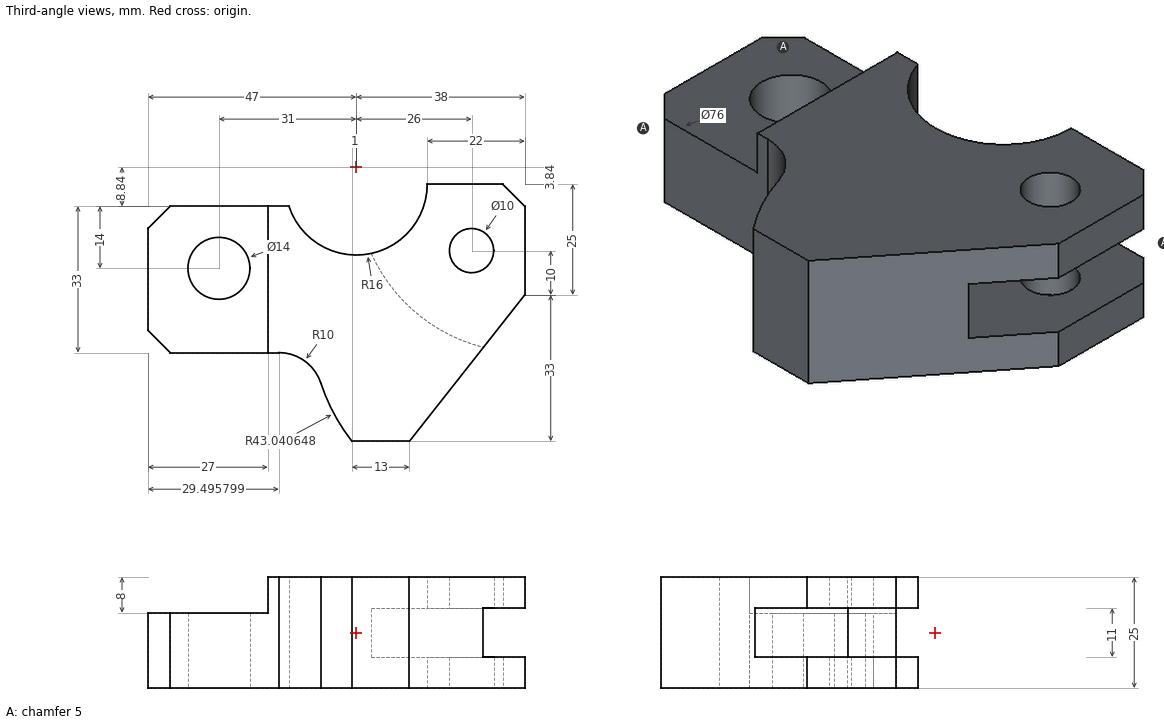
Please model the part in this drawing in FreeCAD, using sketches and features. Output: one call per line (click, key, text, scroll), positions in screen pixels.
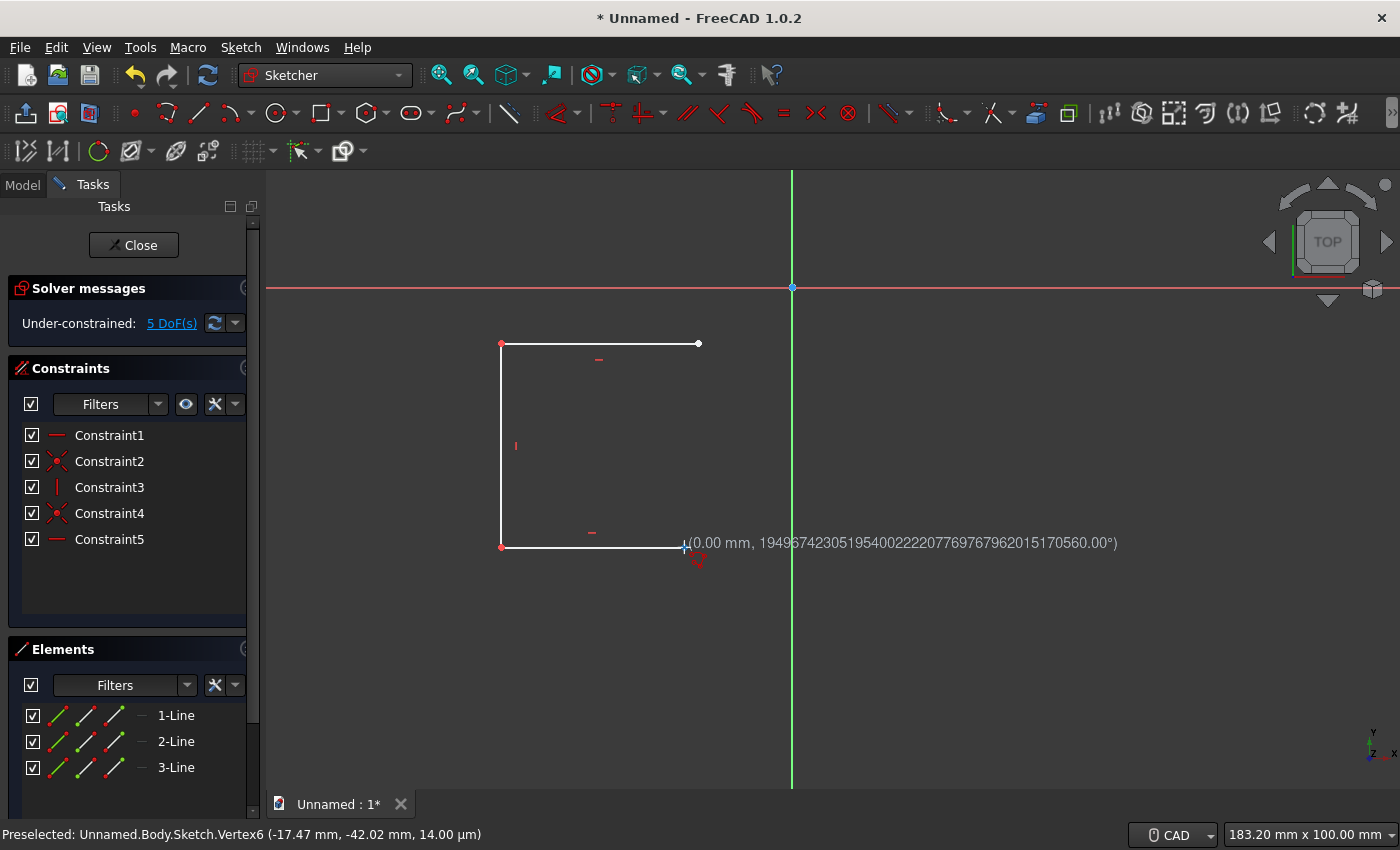
scroll(786, 671, up, 5)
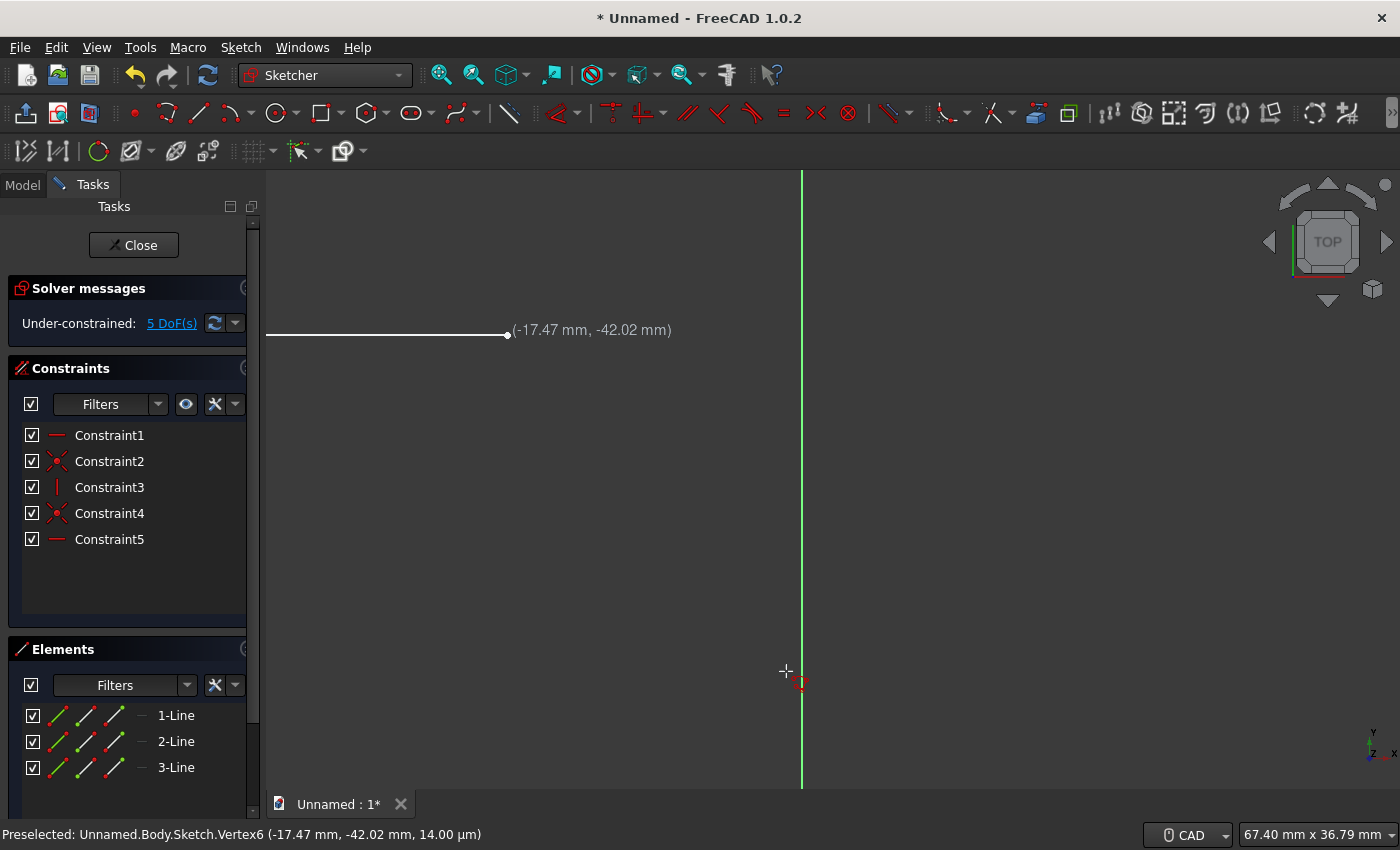
click(785, 669)
click(1004, 669)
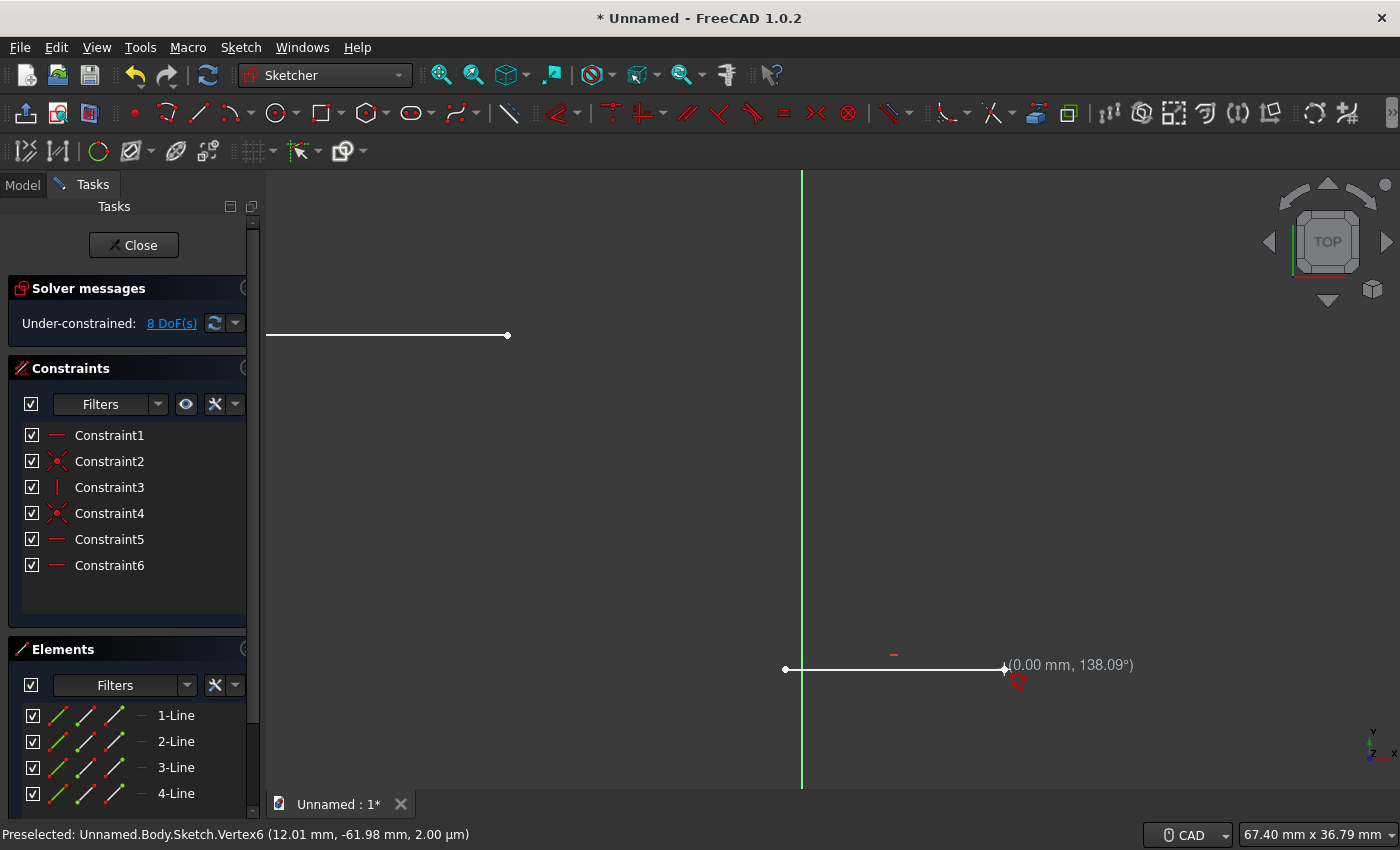
scroll(787, 672, down, 5)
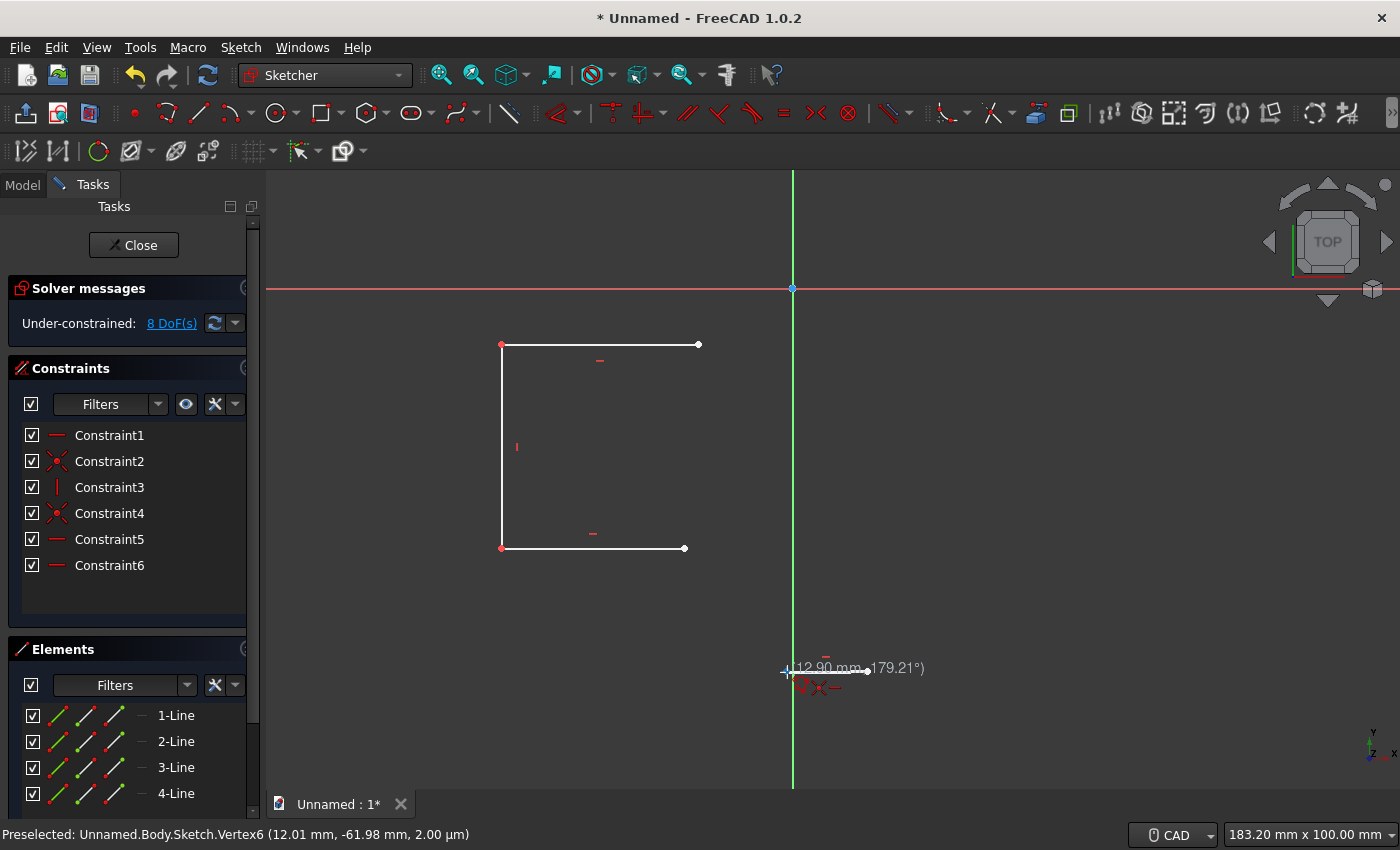
click(1028, 467)
click(1028, 312)
click(892, 312)
right_click(892, 312)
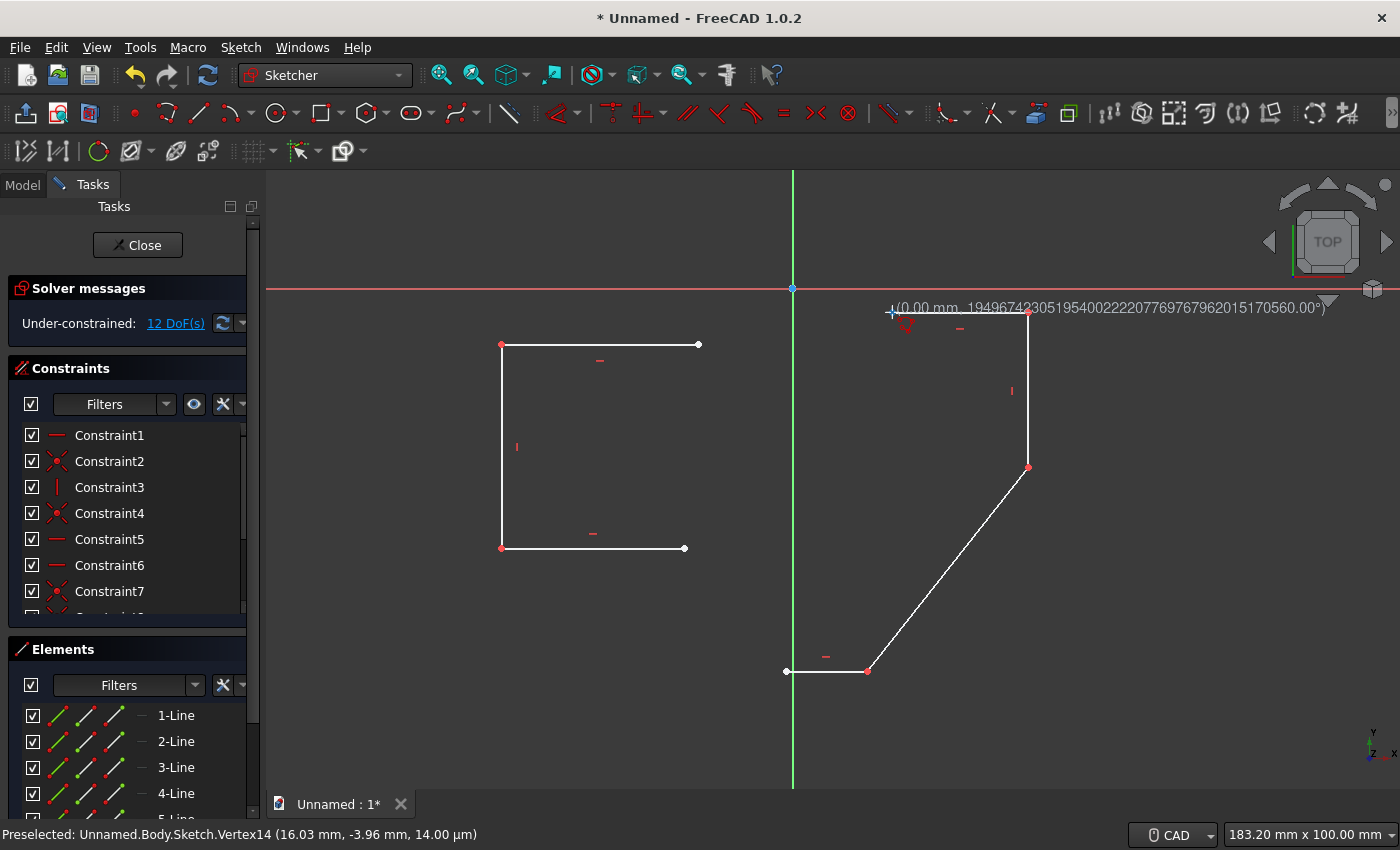
click(254, 114)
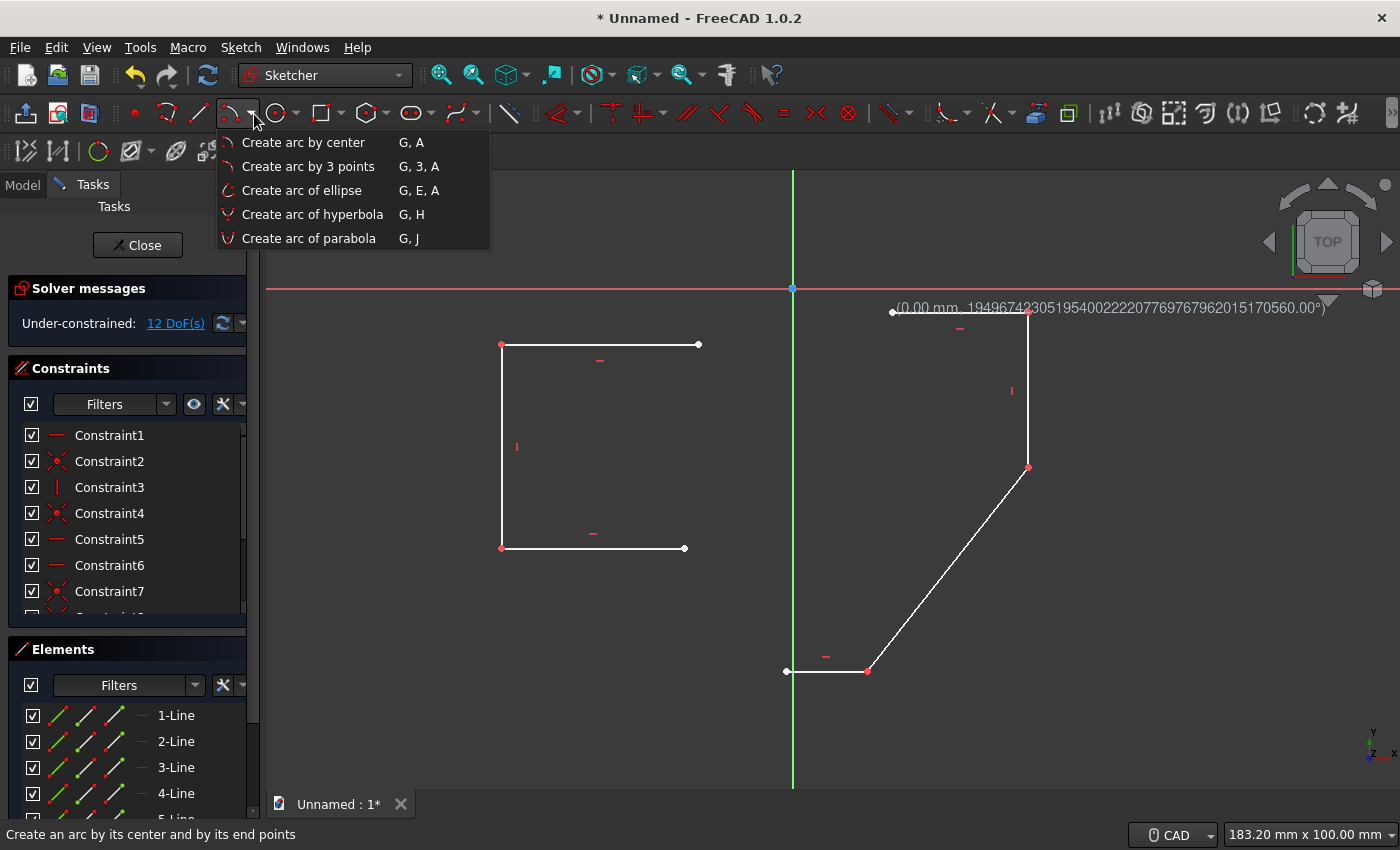
click(354, 166)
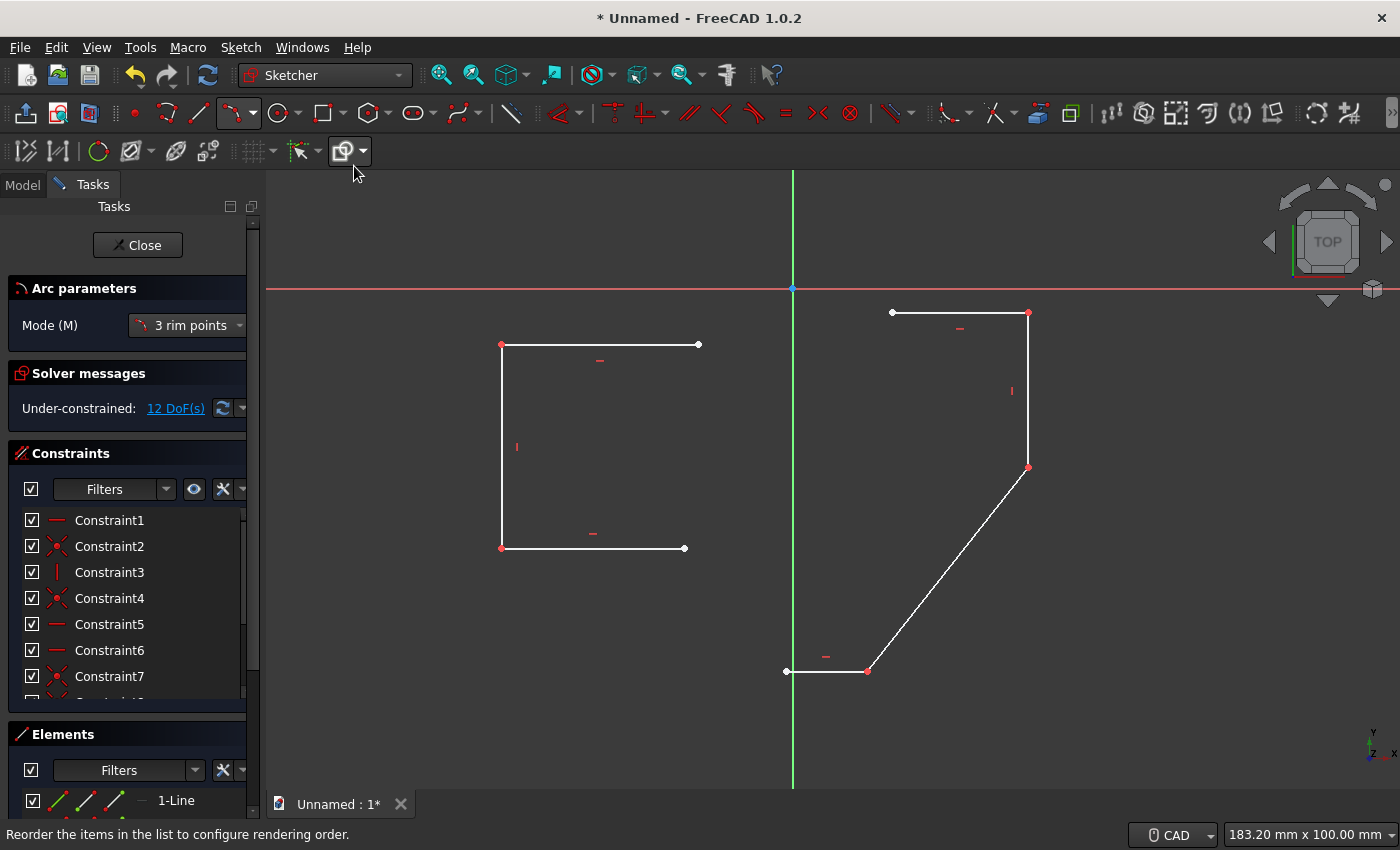
click(685, 549)
click(743, 590)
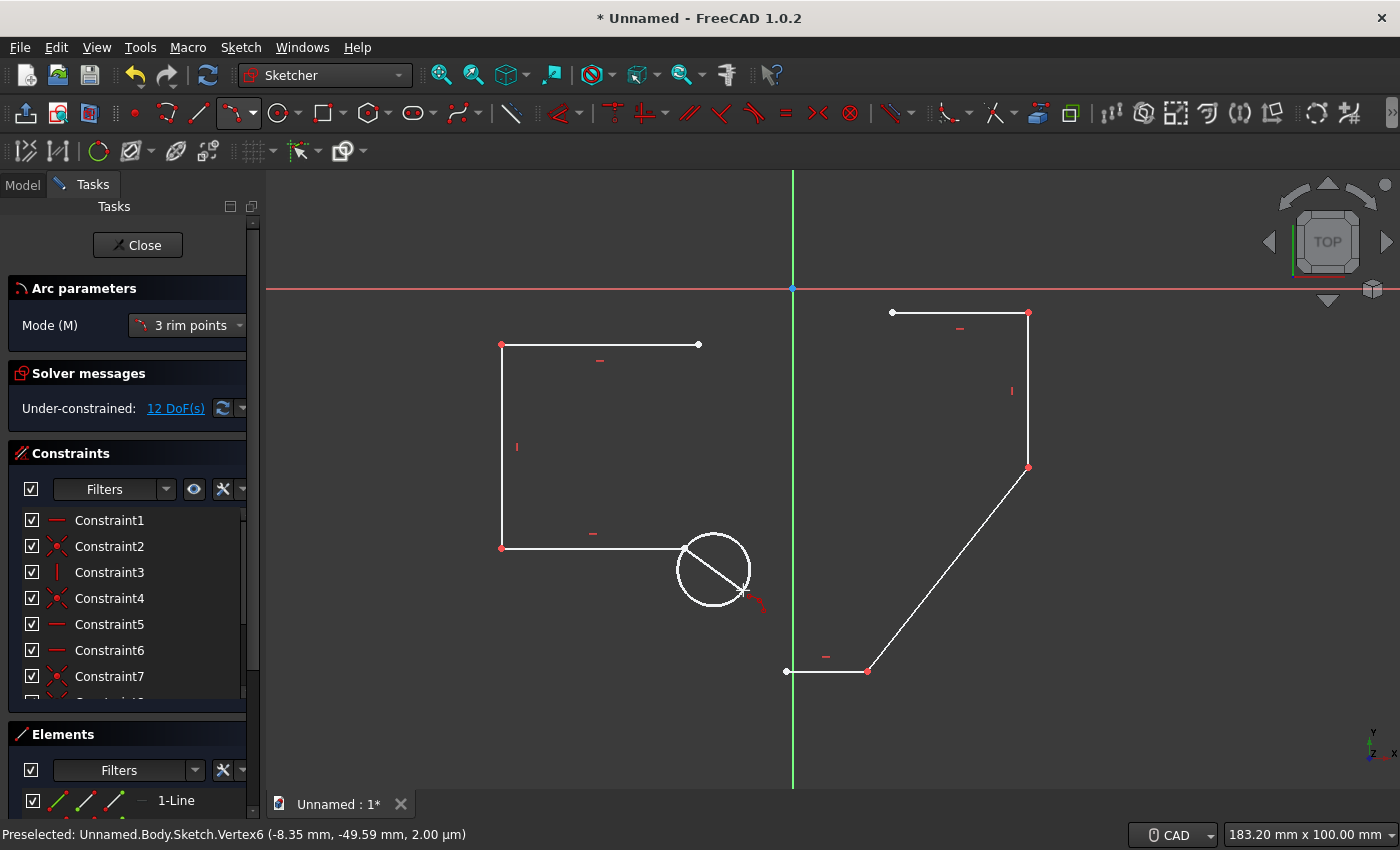
scroll(721, 559, up, 2)